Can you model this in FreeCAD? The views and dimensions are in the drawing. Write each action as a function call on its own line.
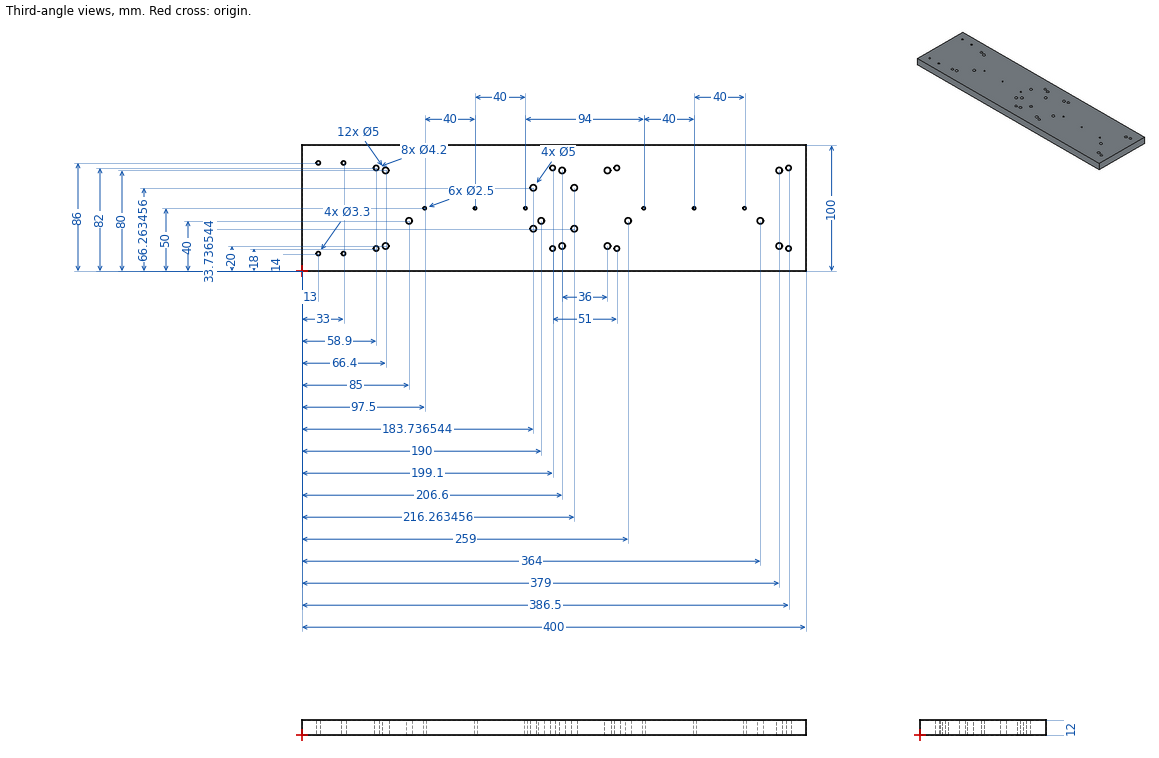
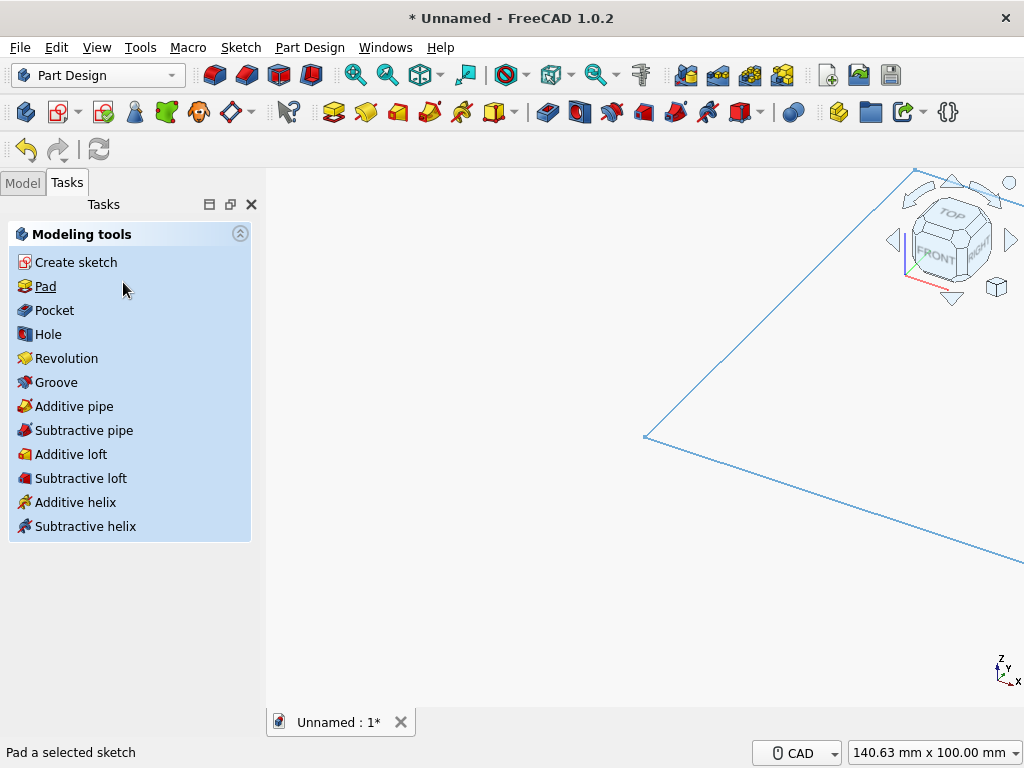
click(334, 112)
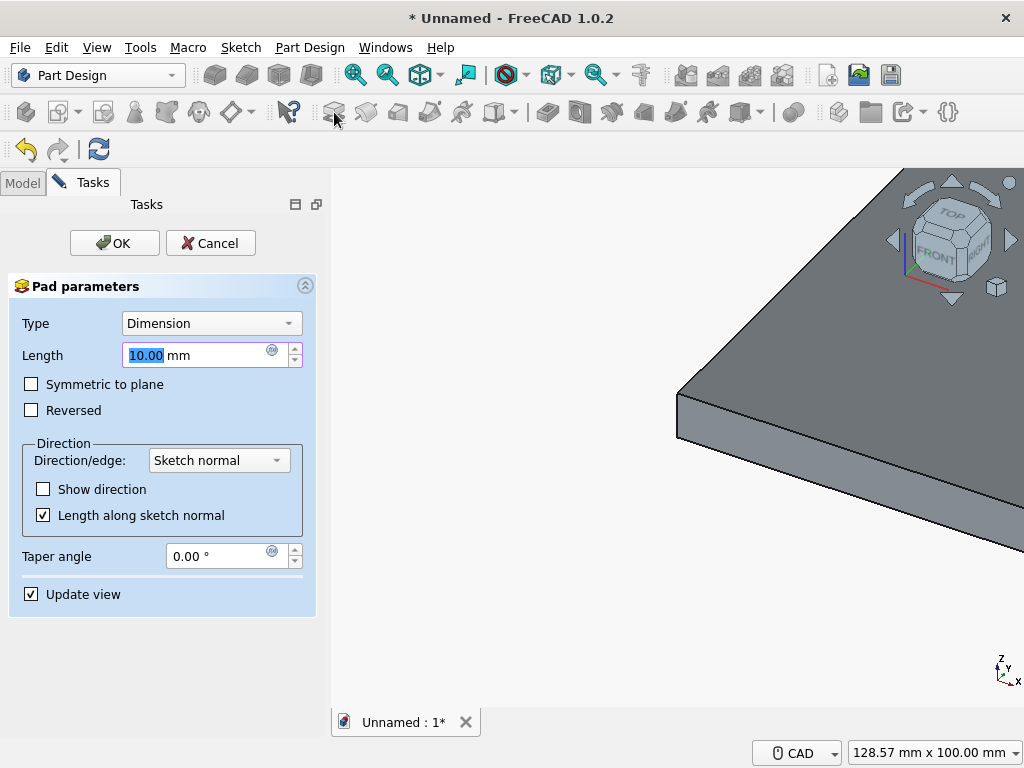
text(12)
key(Tab)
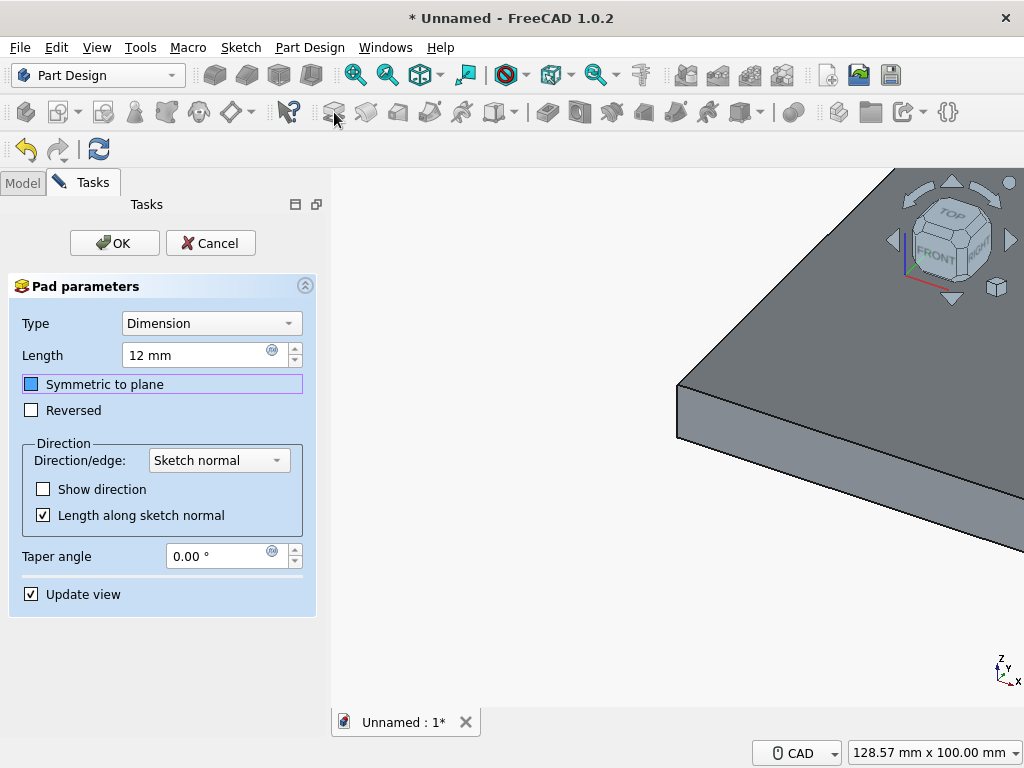
click(115, 243)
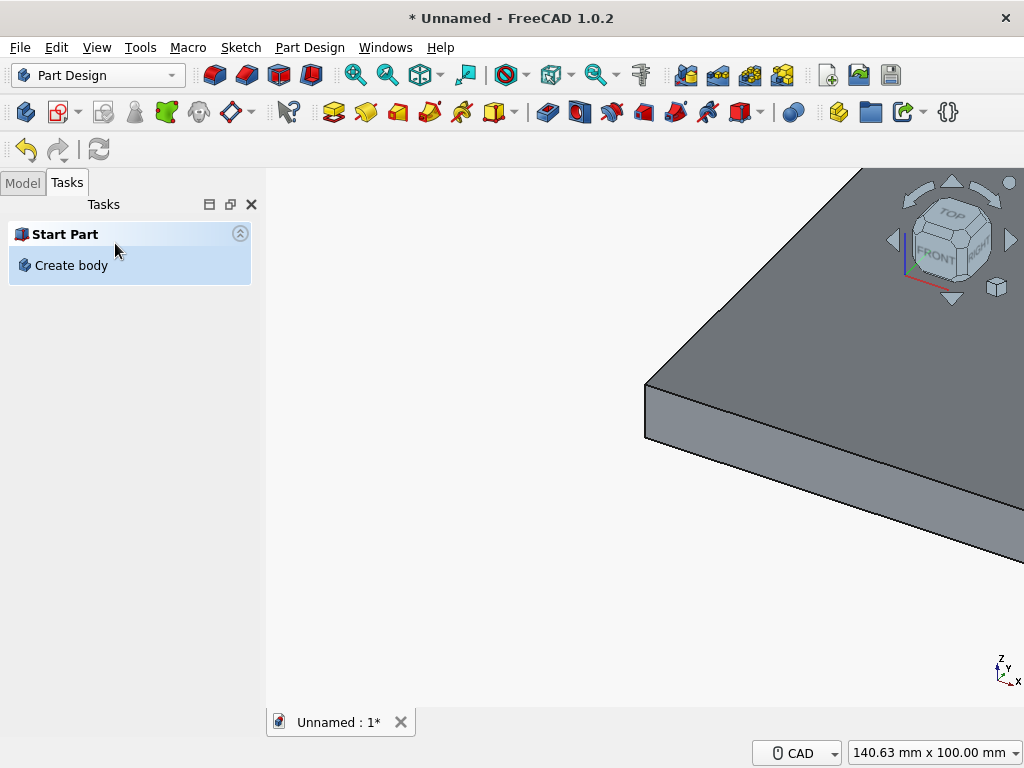
click(356, 76)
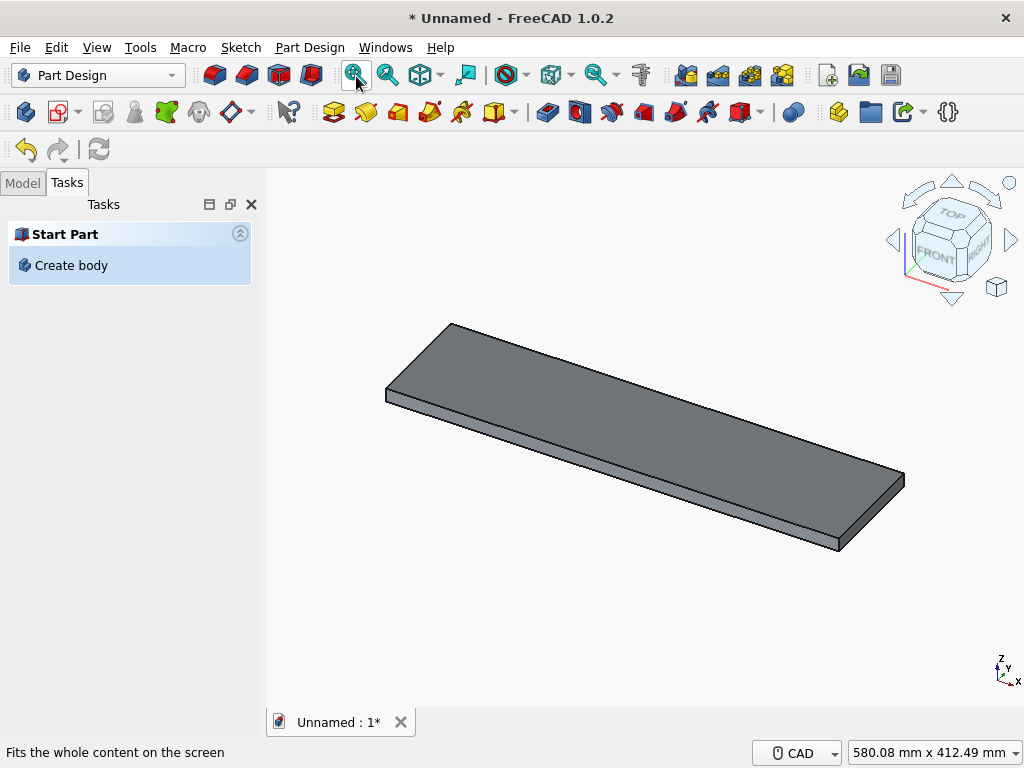
click(774, 473)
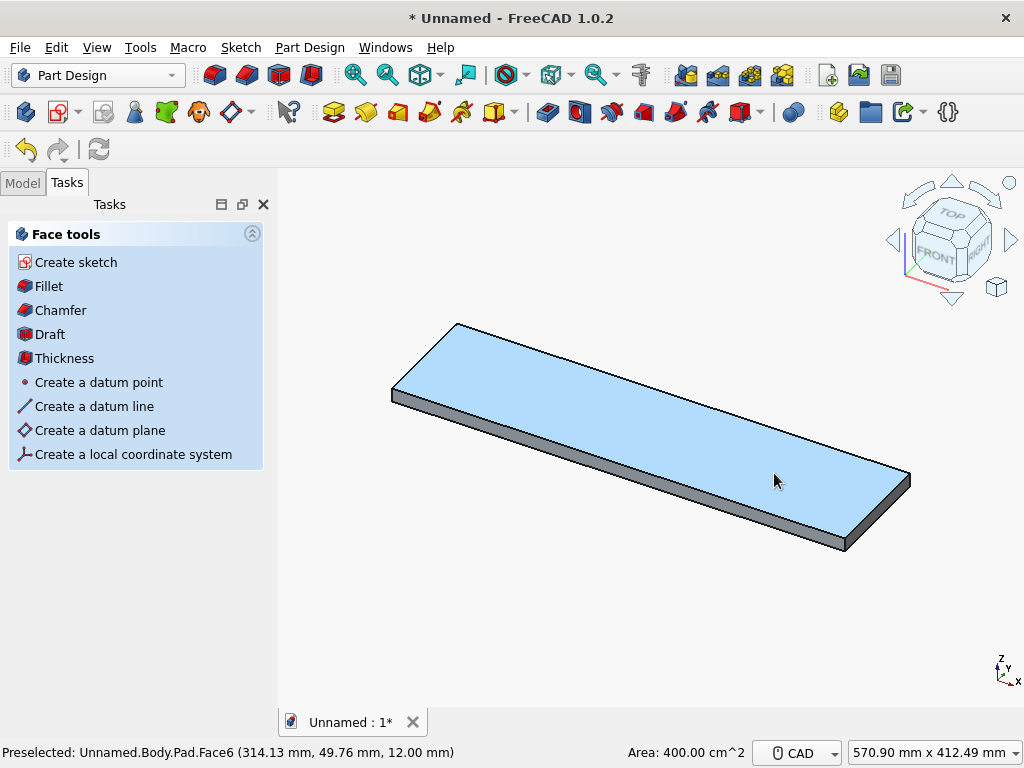
click(58, 112)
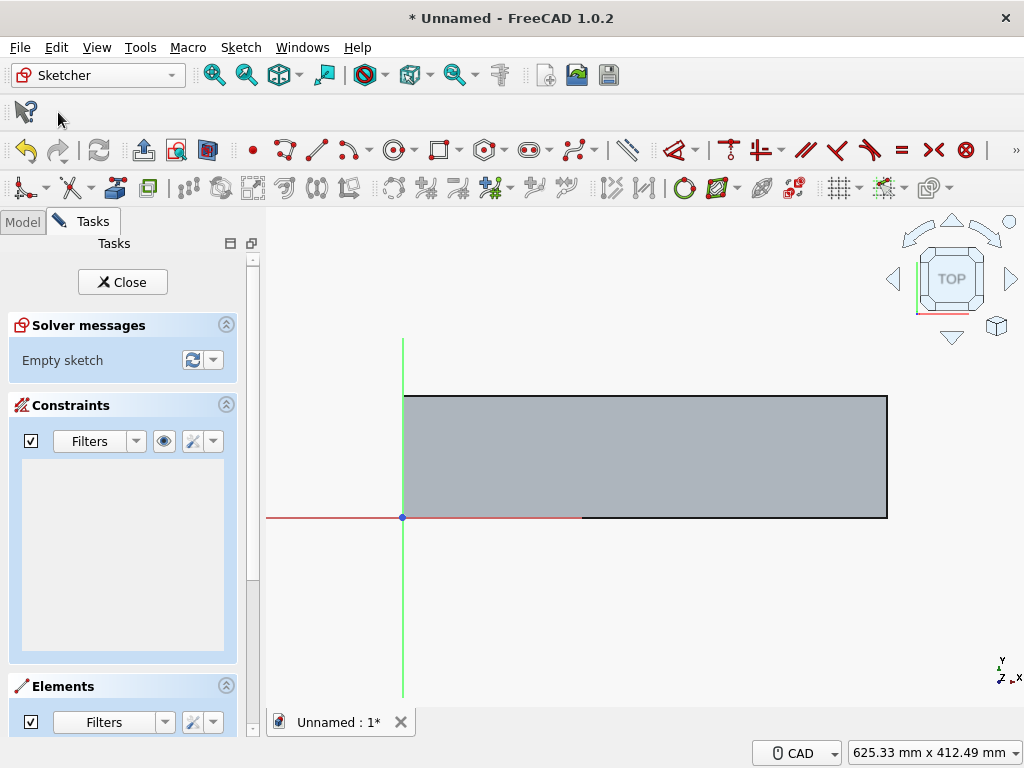
scroll(335, 469, up, 5)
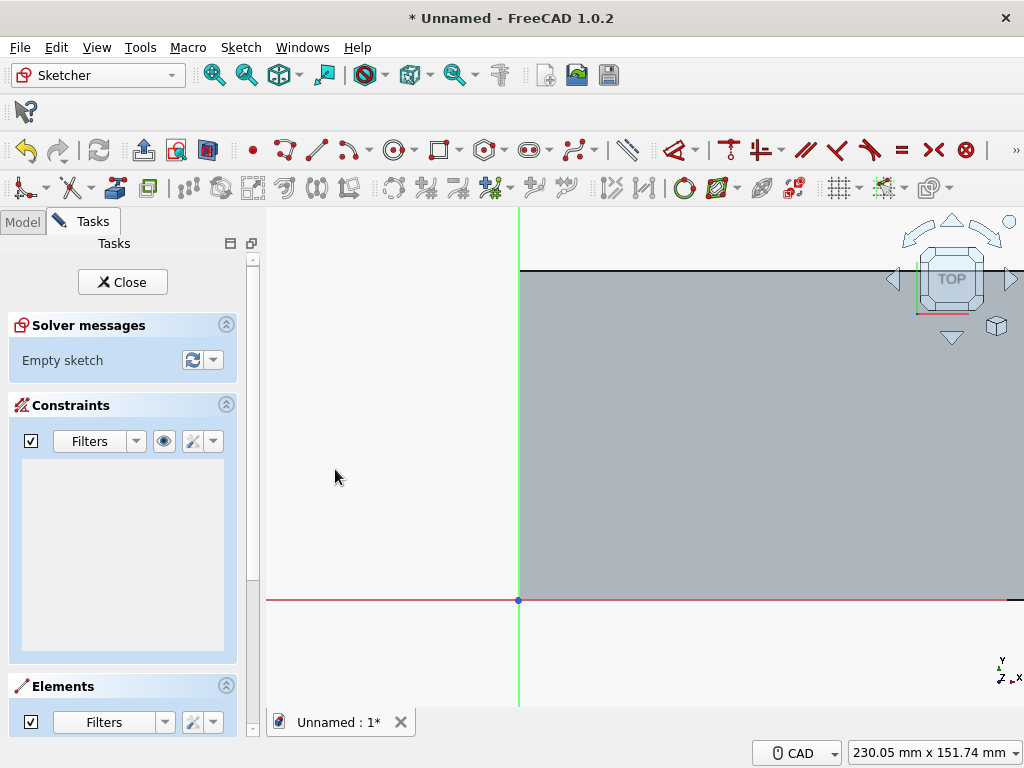
click(394, 150)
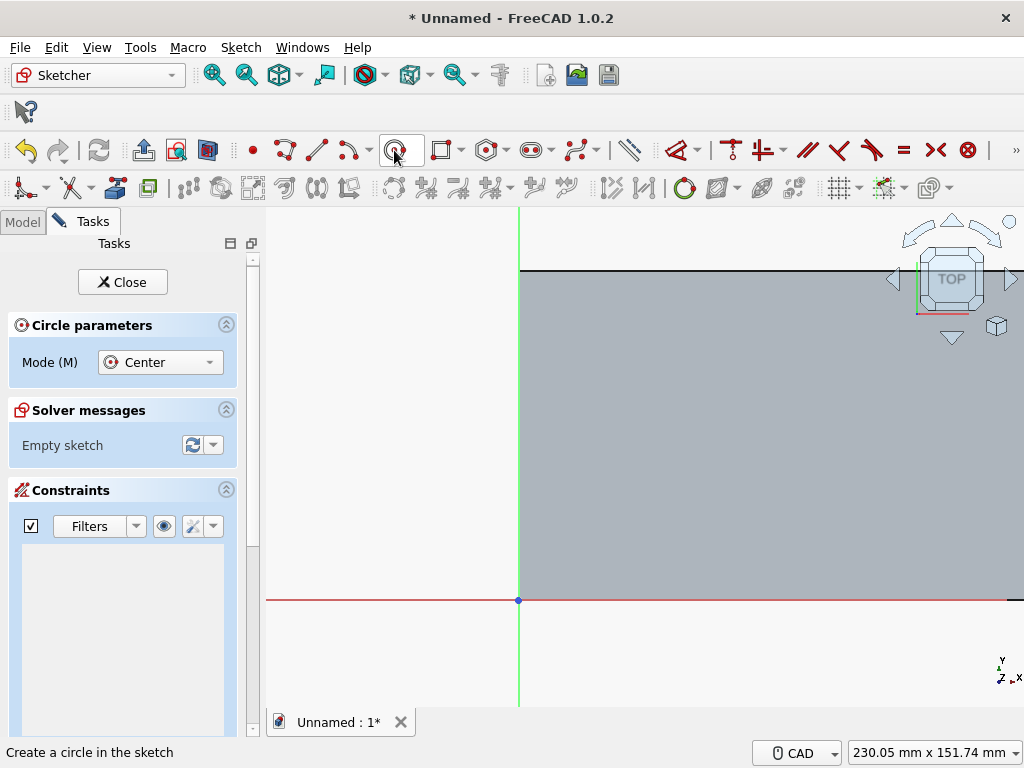
scroll(561, 554, up, 8)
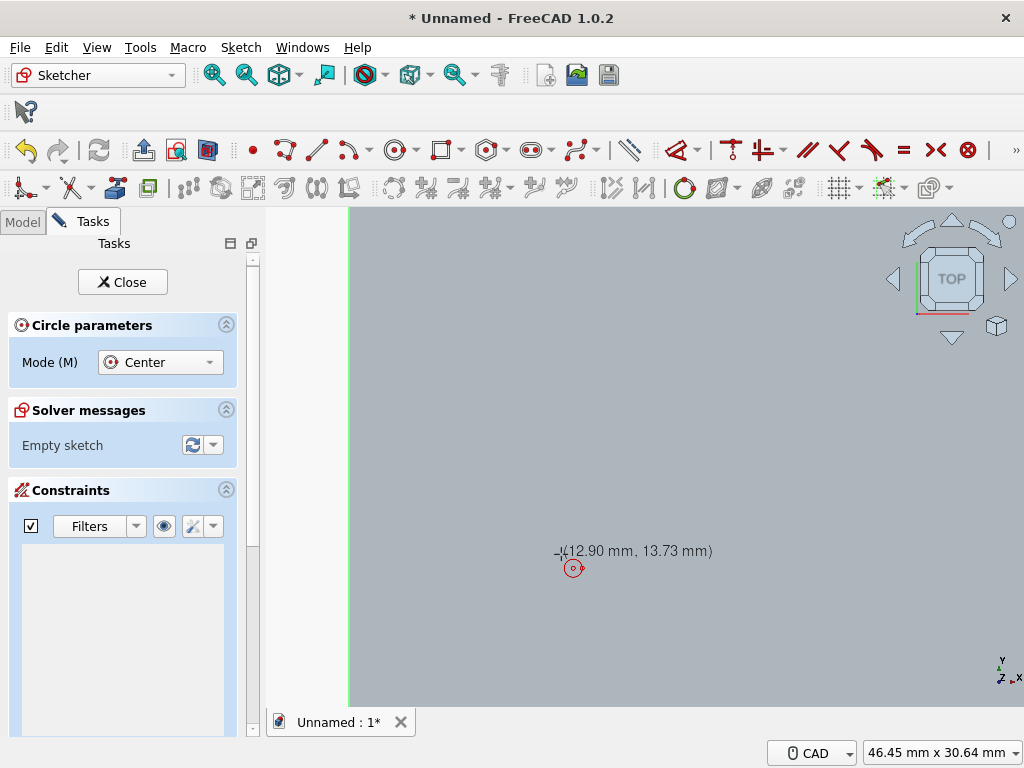
scroll(563, 556, down, 8)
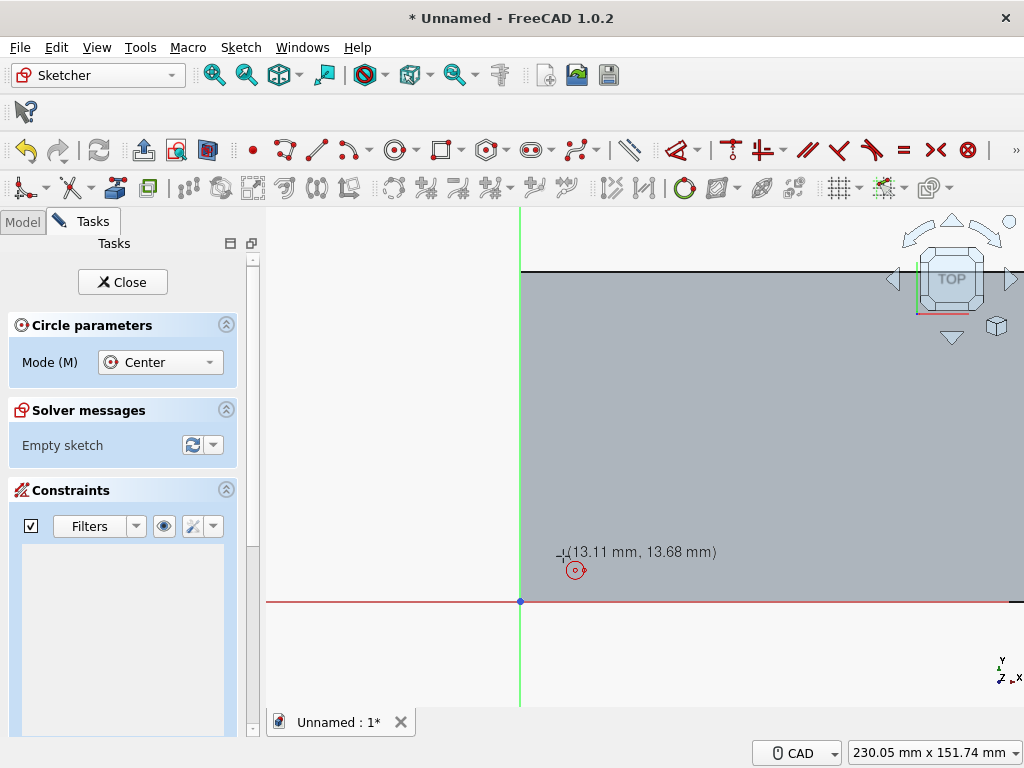
click(563, 556)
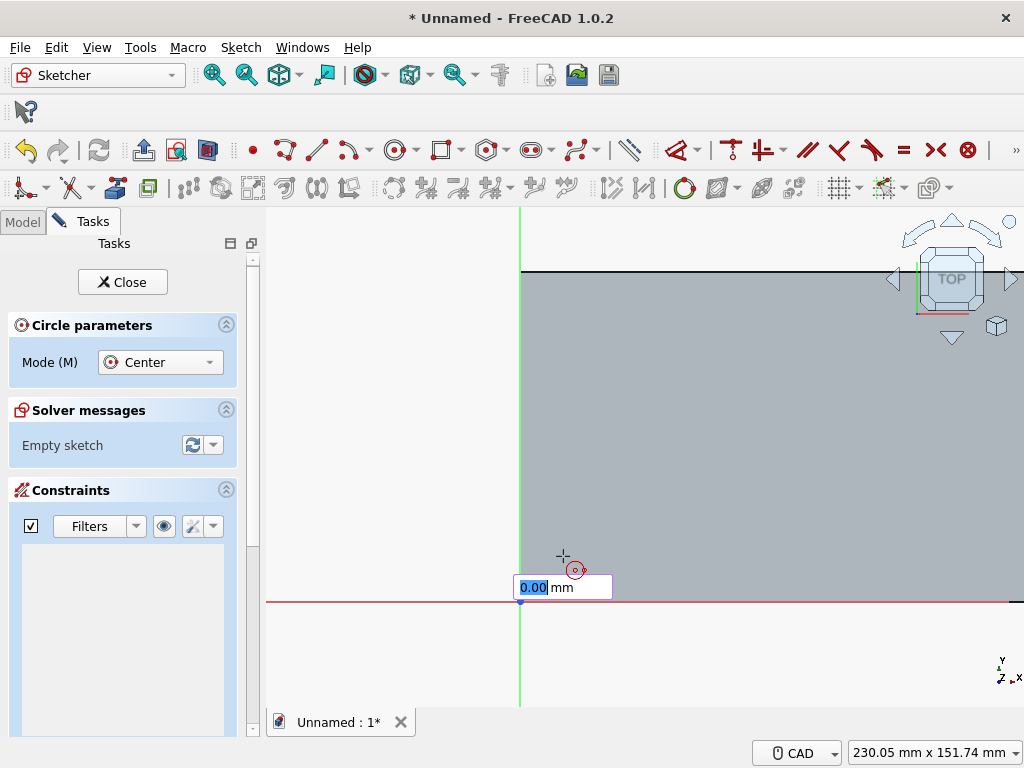
scroll(567, 552, up, 6)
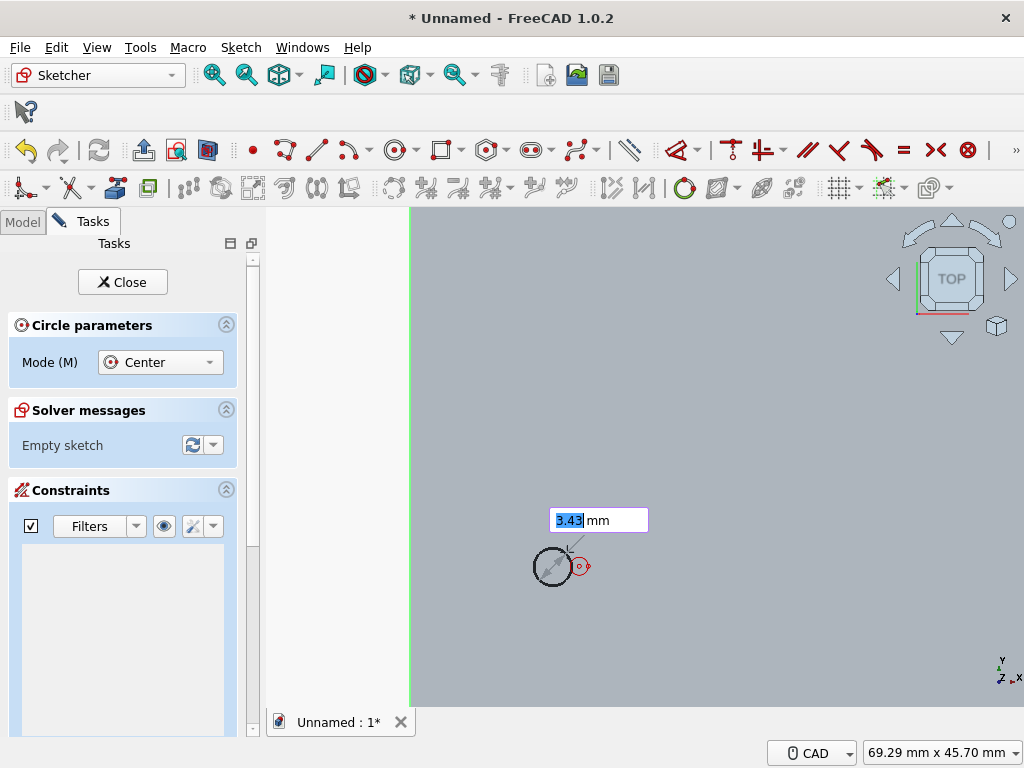
click(565, 550)